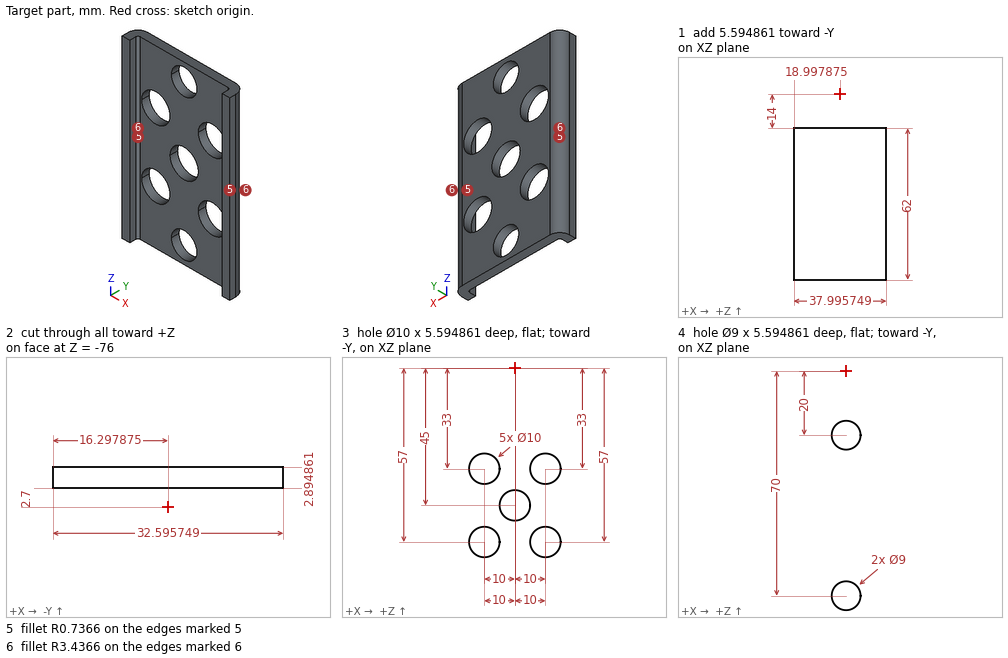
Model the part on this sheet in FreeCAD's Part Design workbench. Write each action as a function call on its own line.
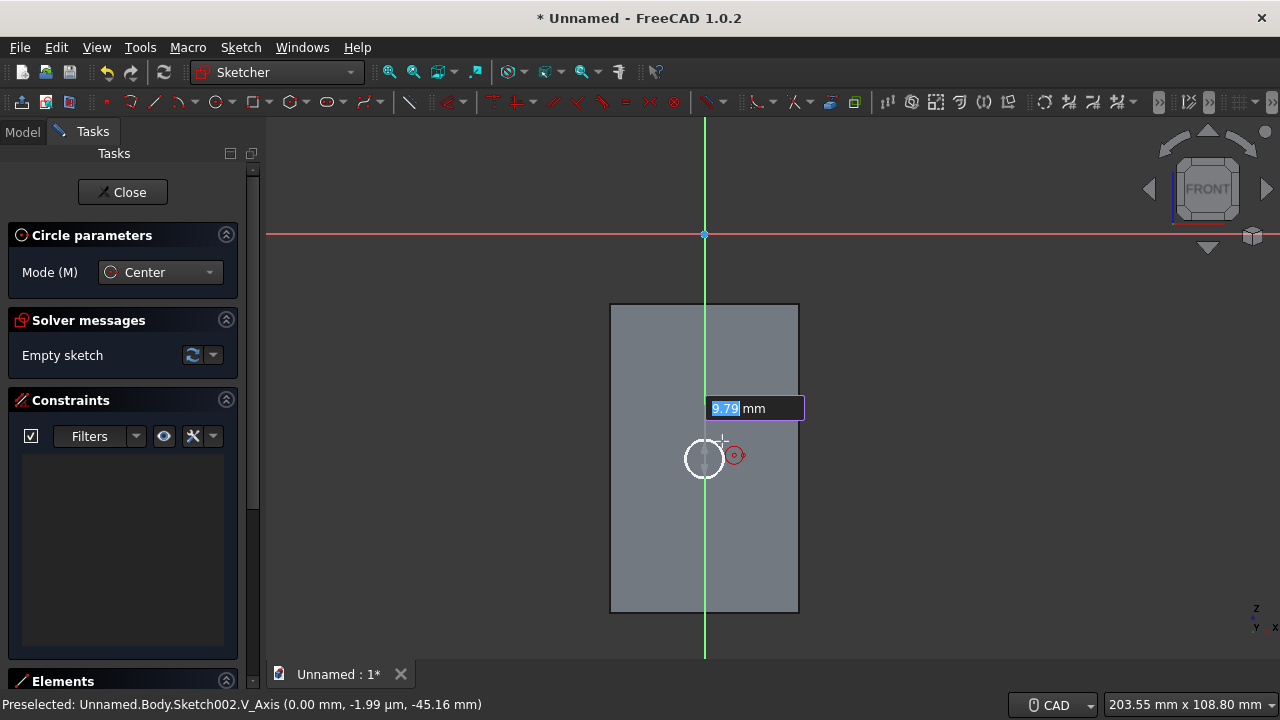
text(10)
key(Return)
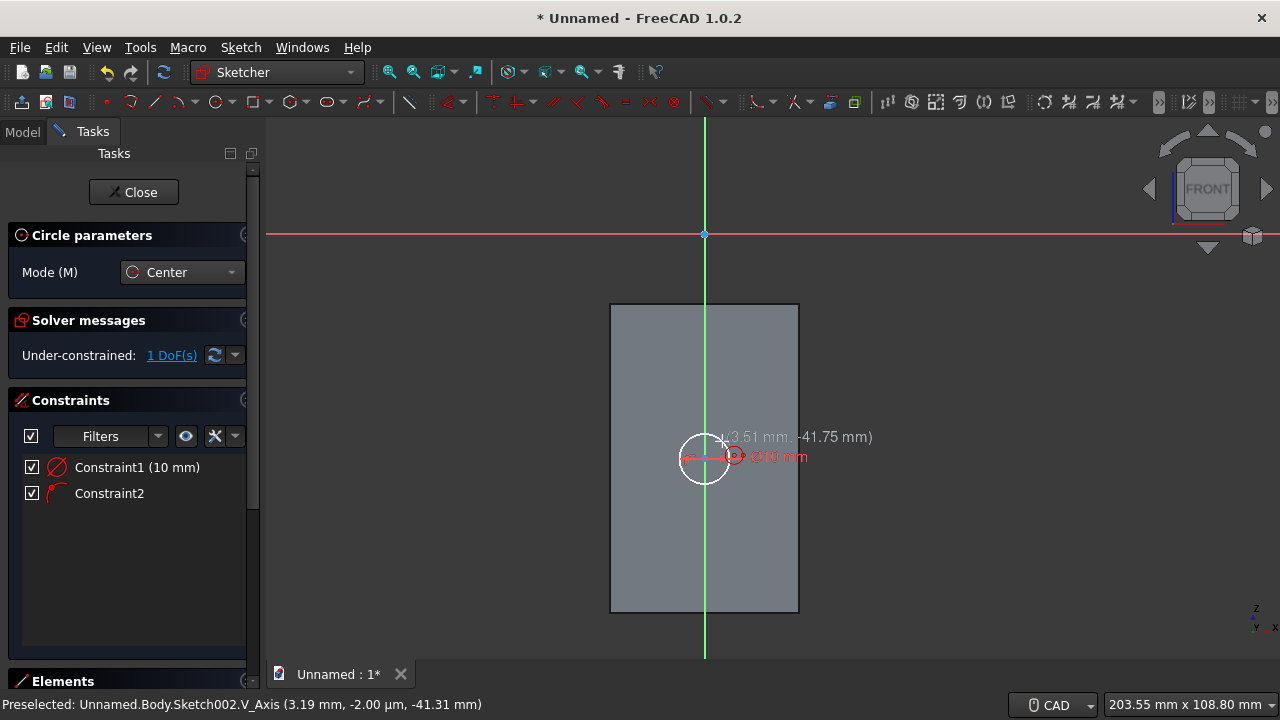
click(655, 518)
move(672, 500)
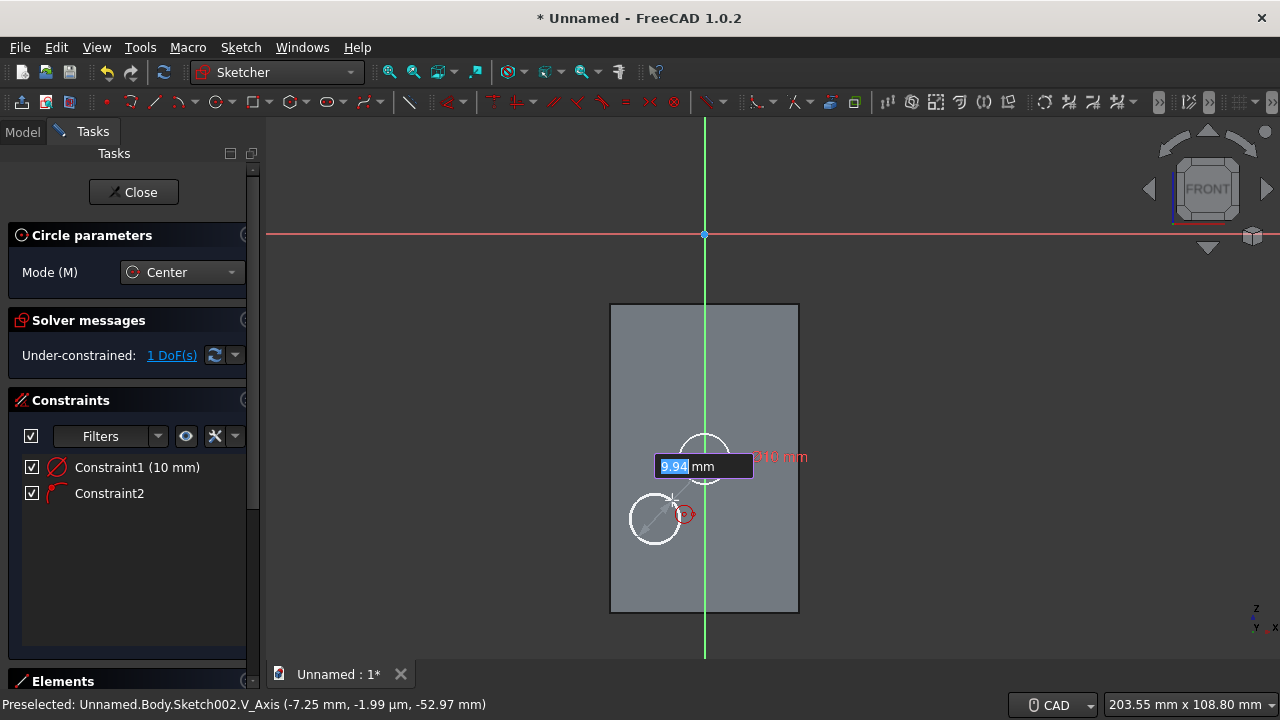
text(10)
key(Return)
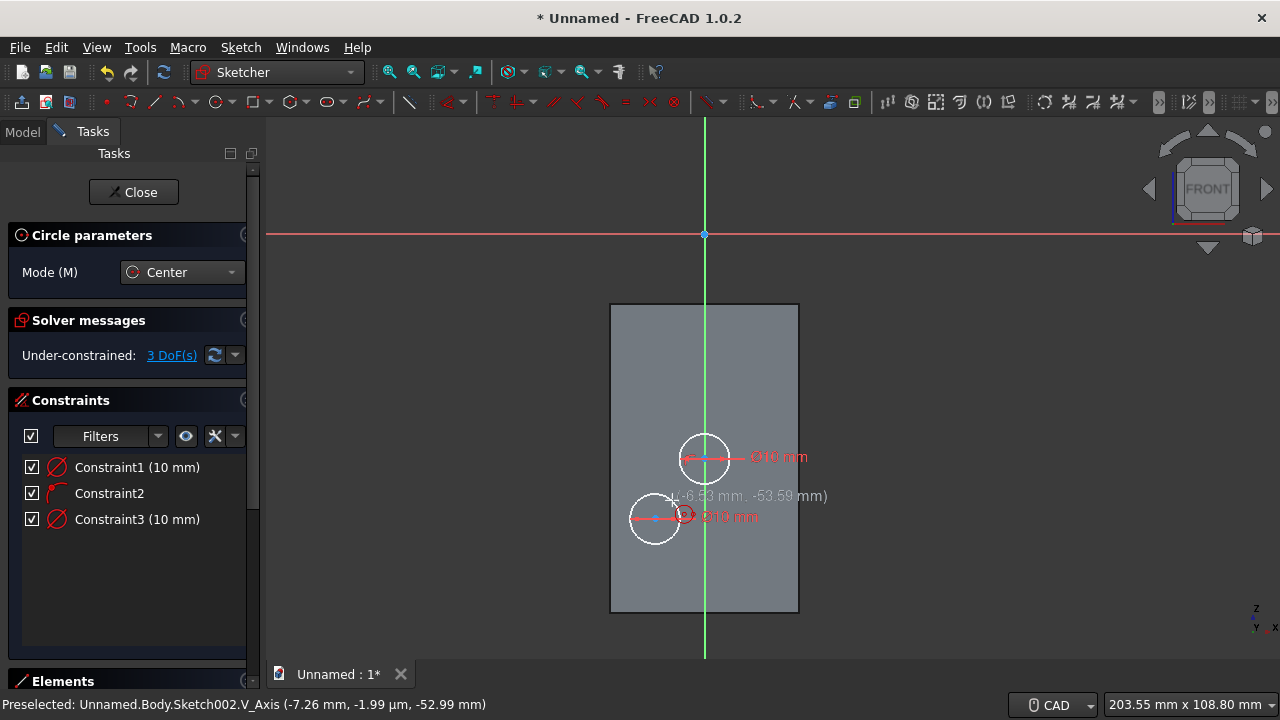
click(655, 398)
move(672, 381)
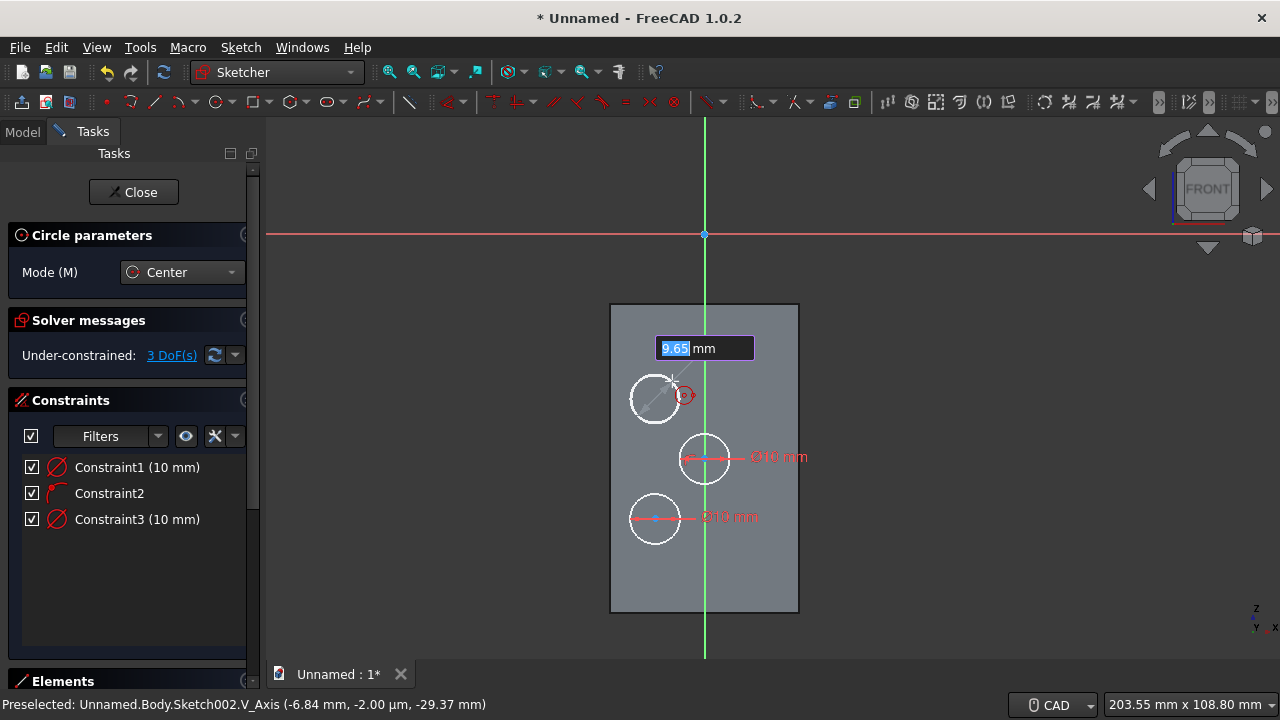
text(10)
key(Return)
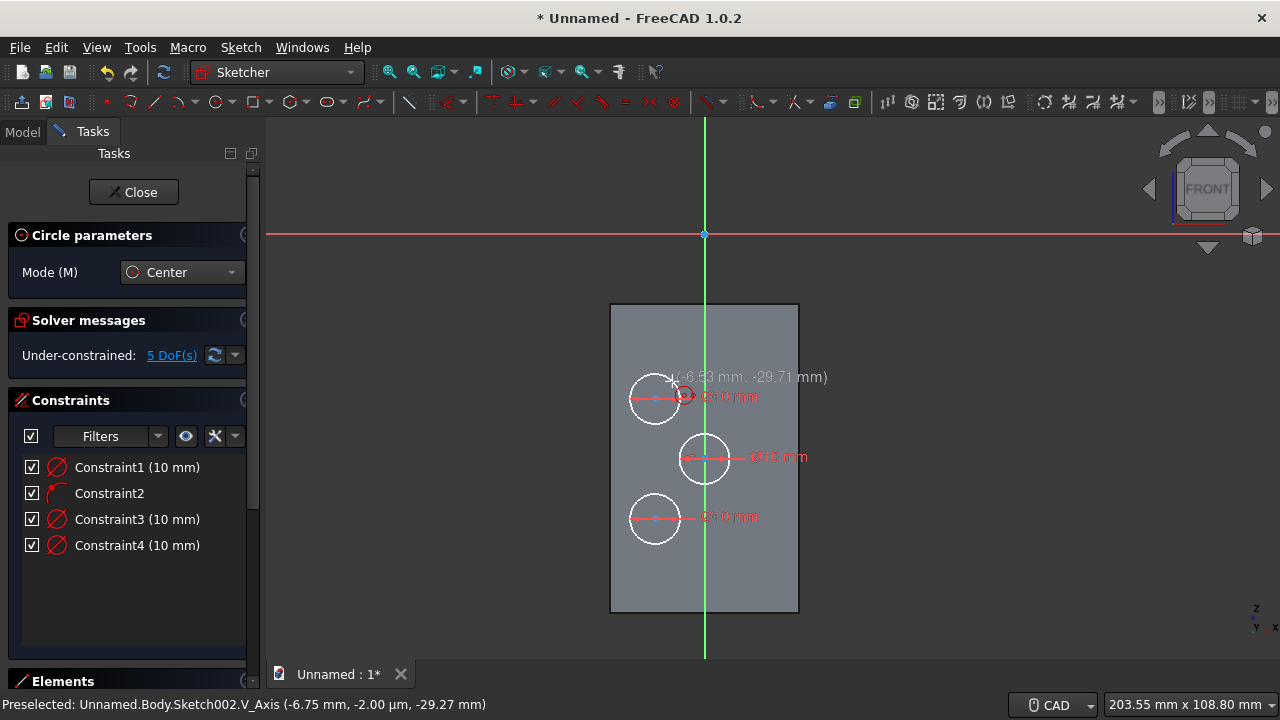
click(754, 398)
move(772, 381)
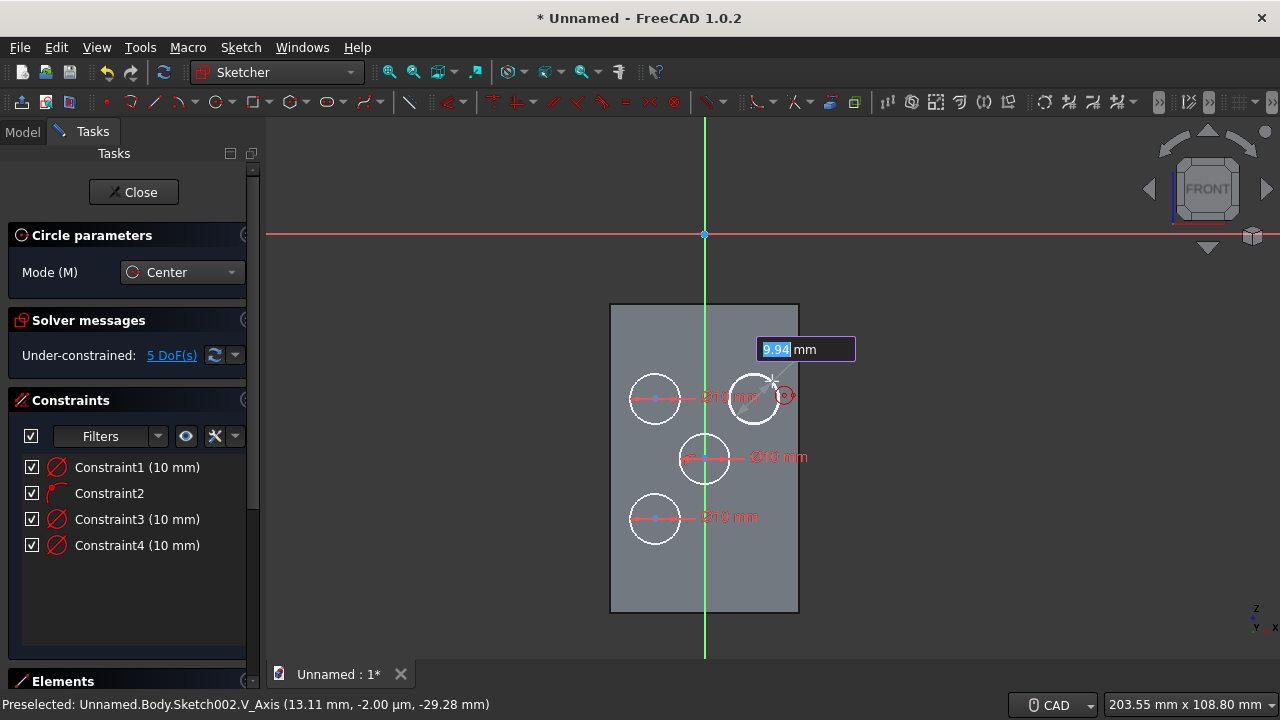
text(10)
key(Return)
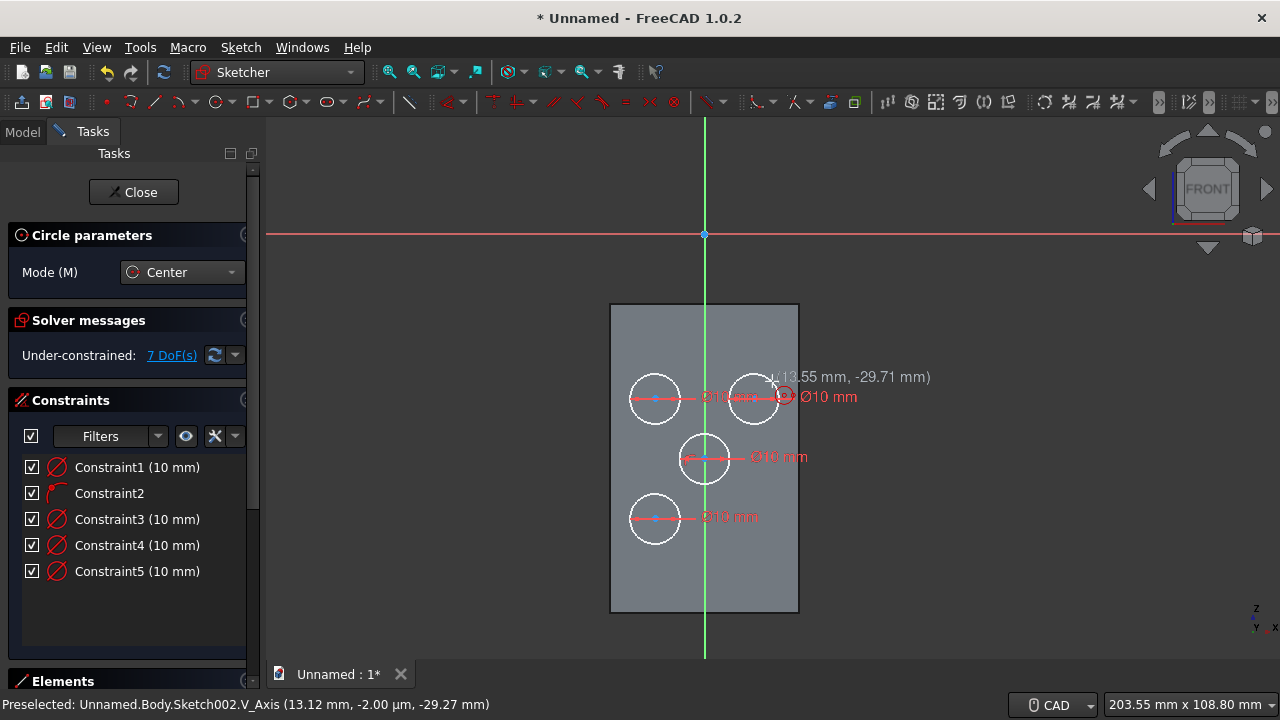
click(754, 518)
move(772, 500)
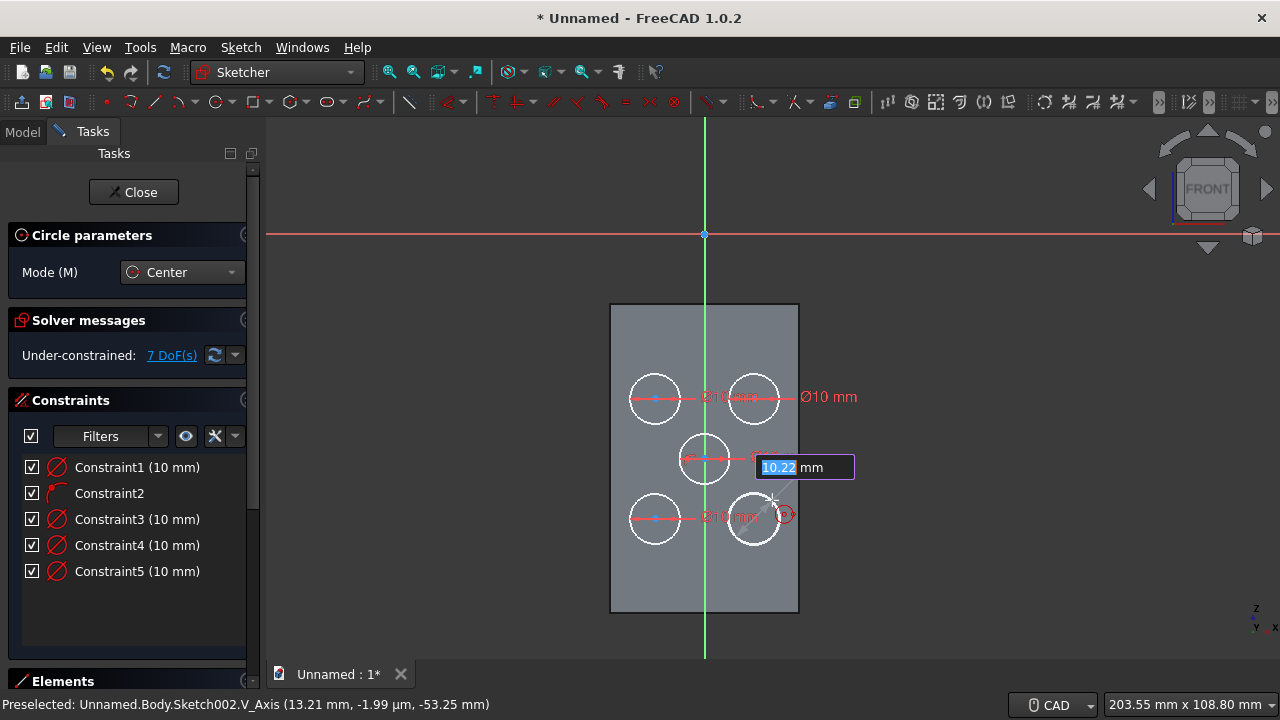
text(10)
key(Return)
key(Escape)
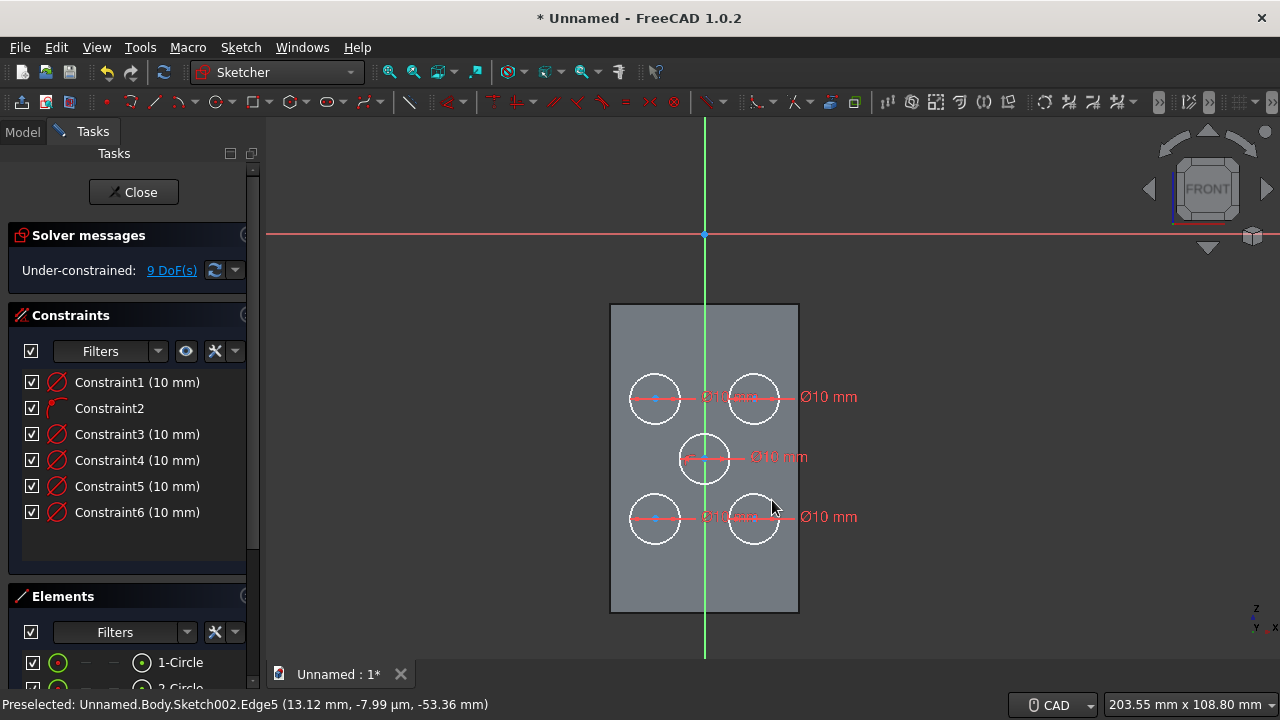
click(448, 102)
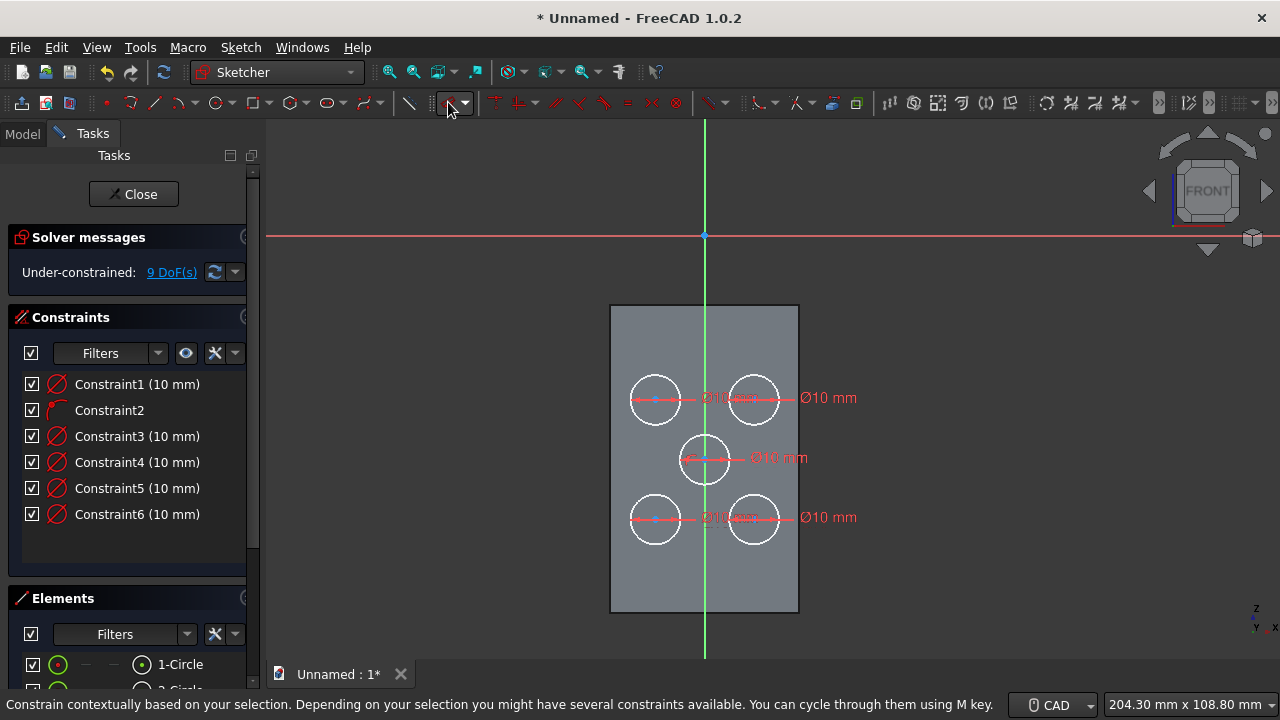
click(705, 460)
click(739, 348)